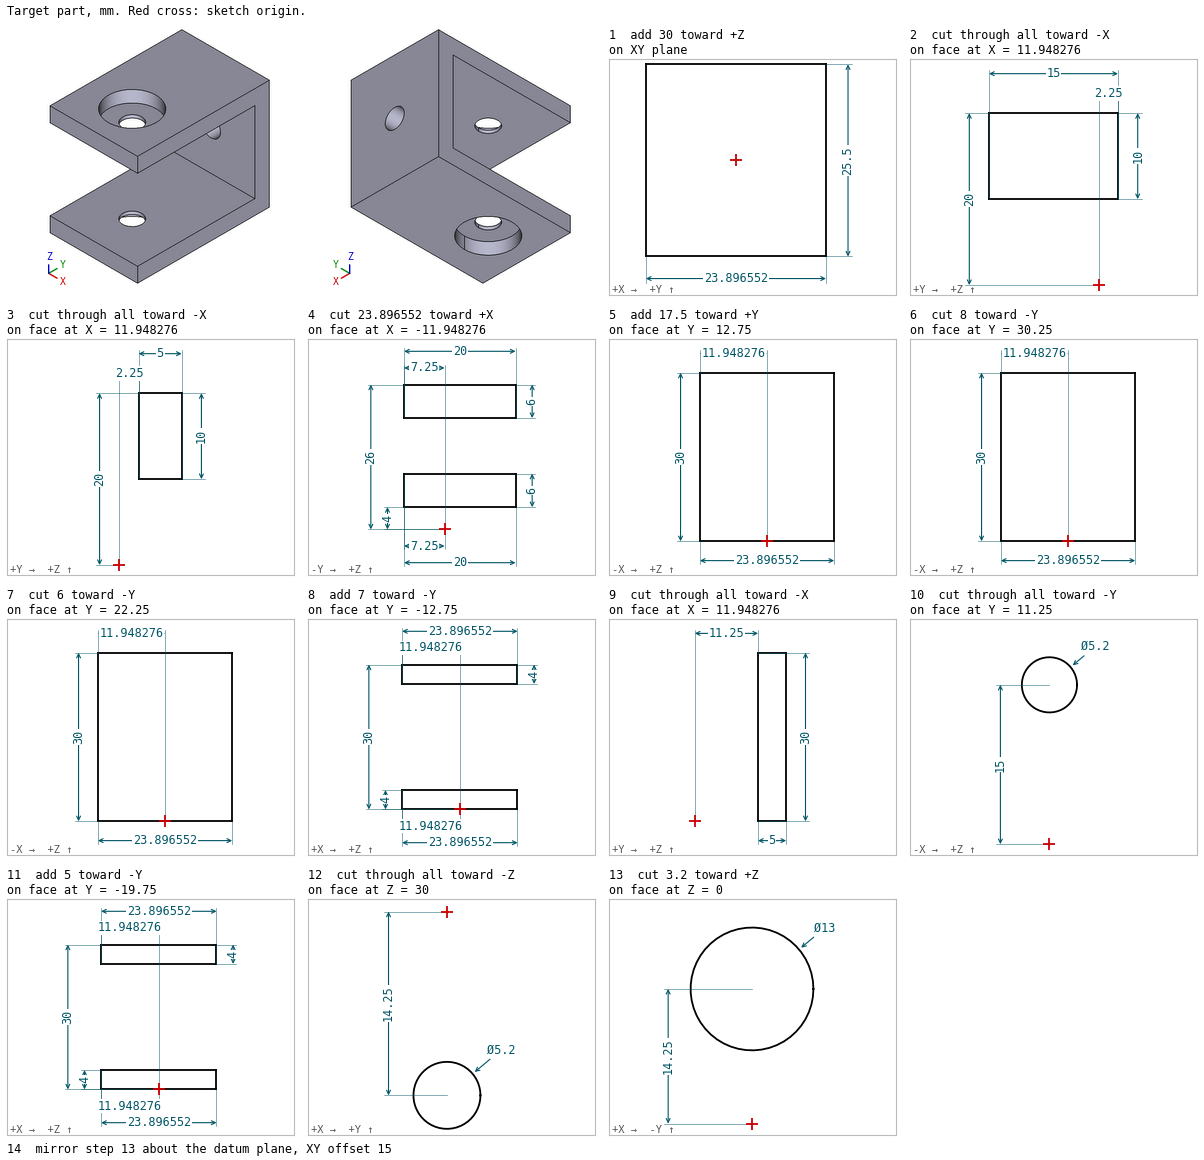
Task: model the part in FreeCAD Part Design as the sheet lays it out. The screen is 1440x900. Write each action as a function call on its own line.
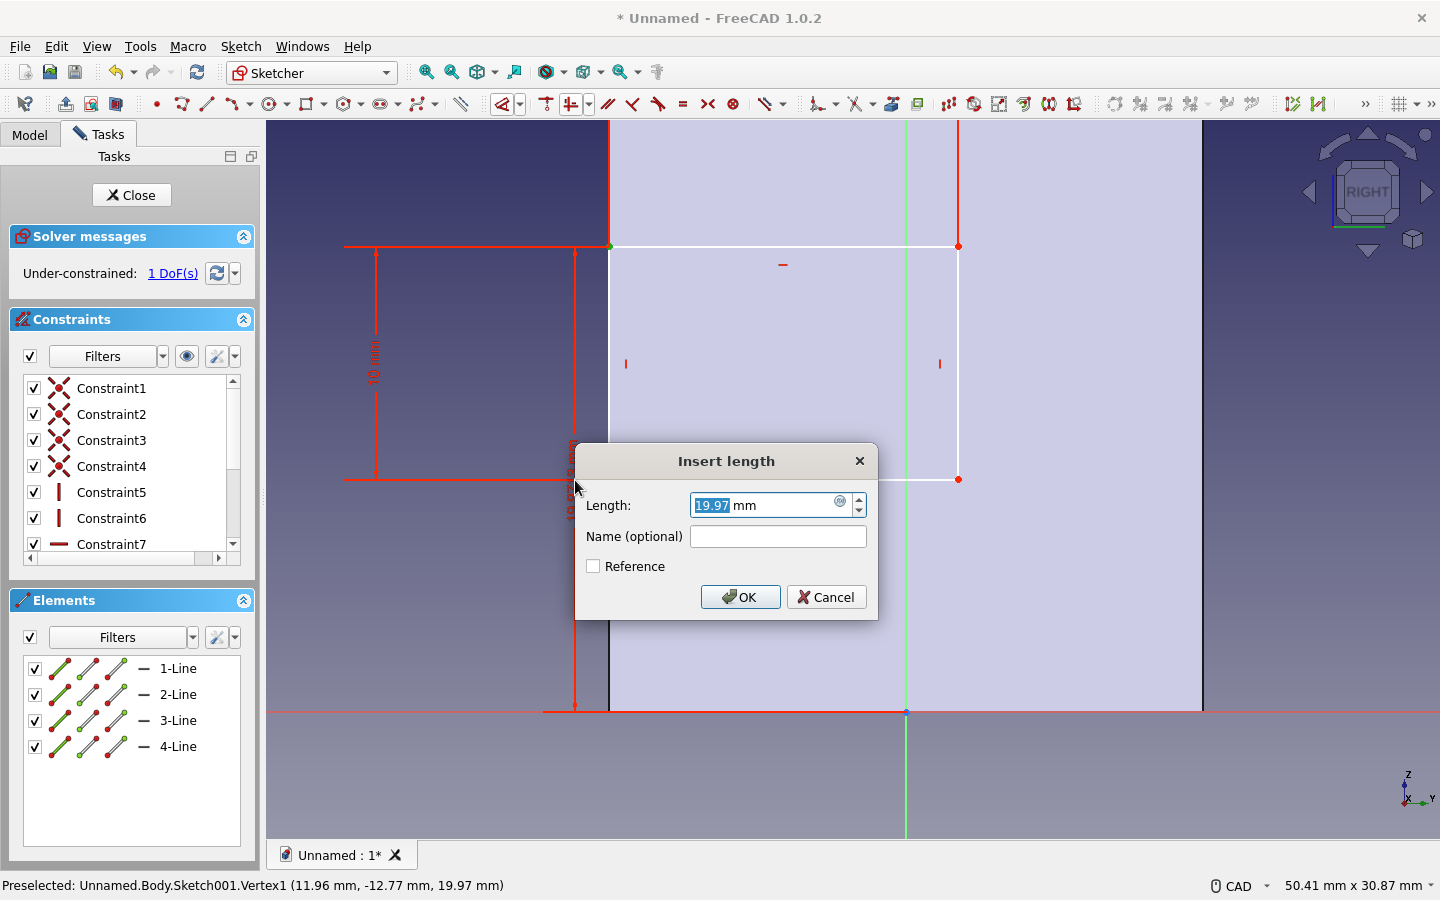
text(20)
key(Return)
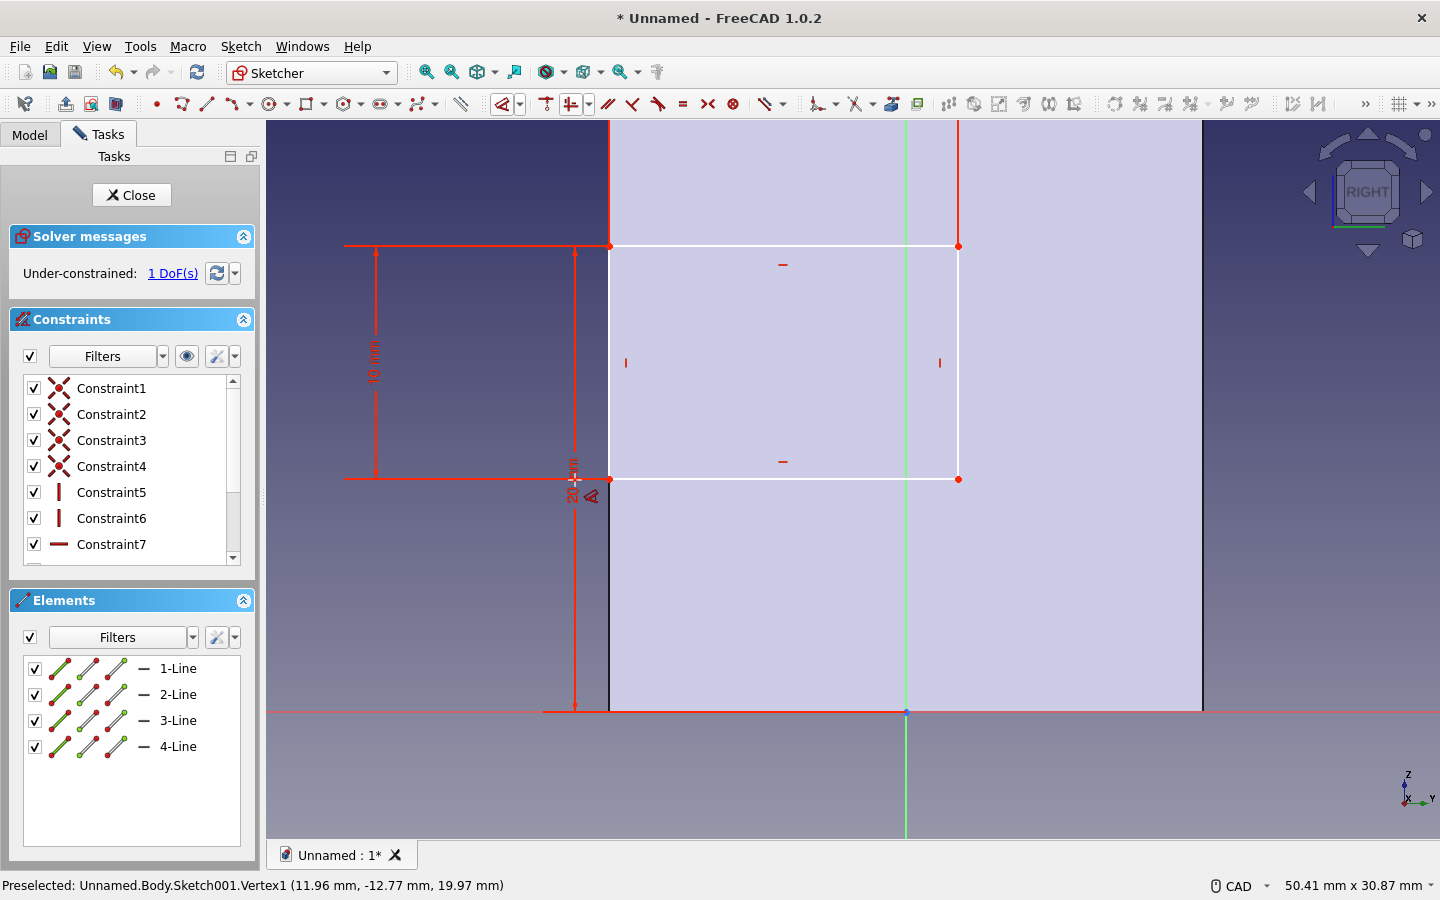
click(958, 479)
click(932, 746)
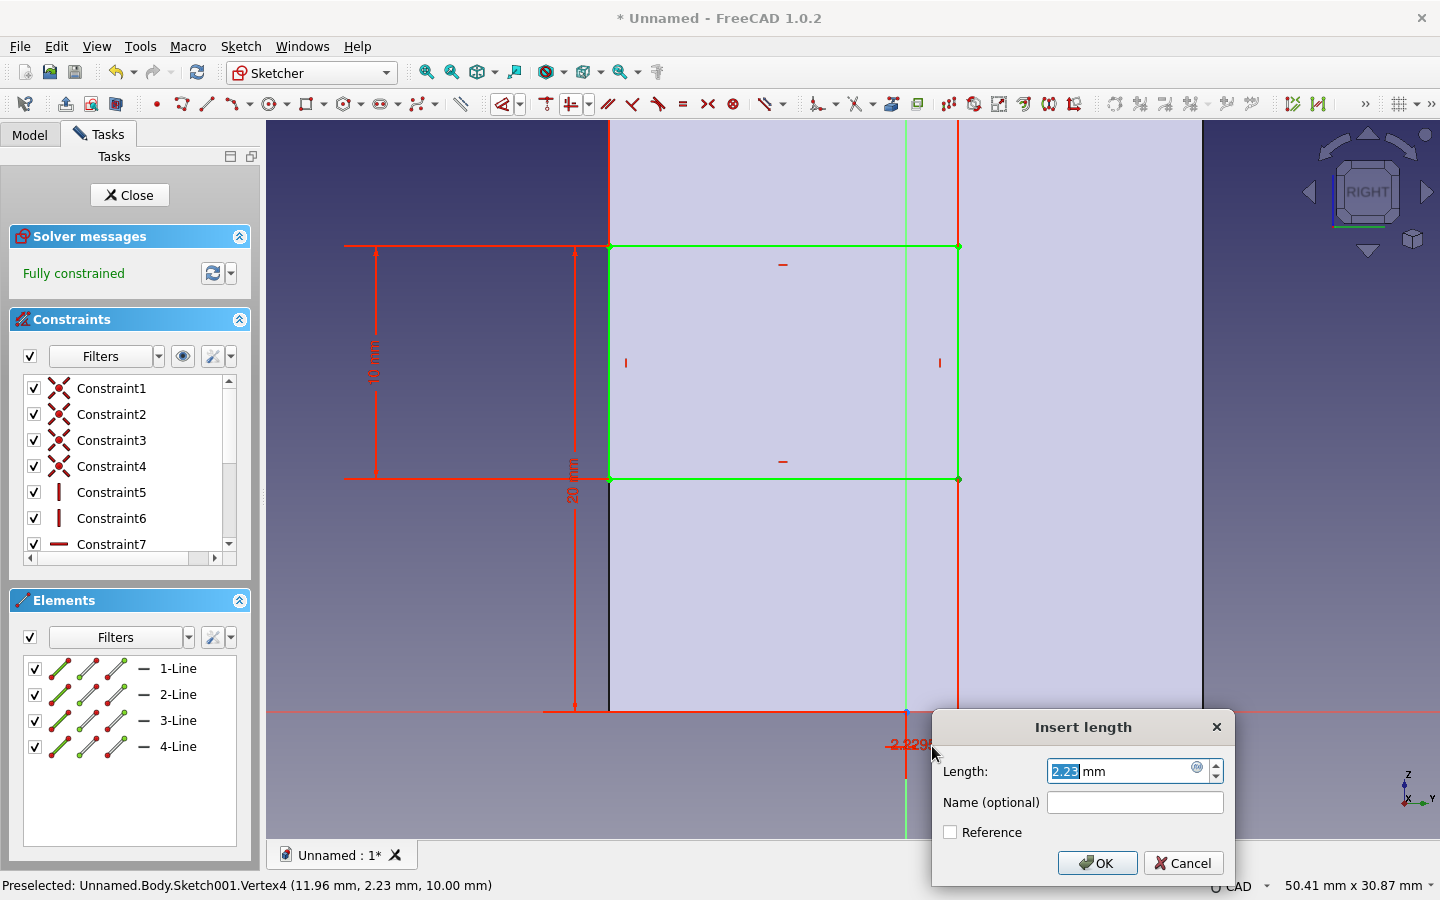
text(2.25)
key(Return)
key(Escape)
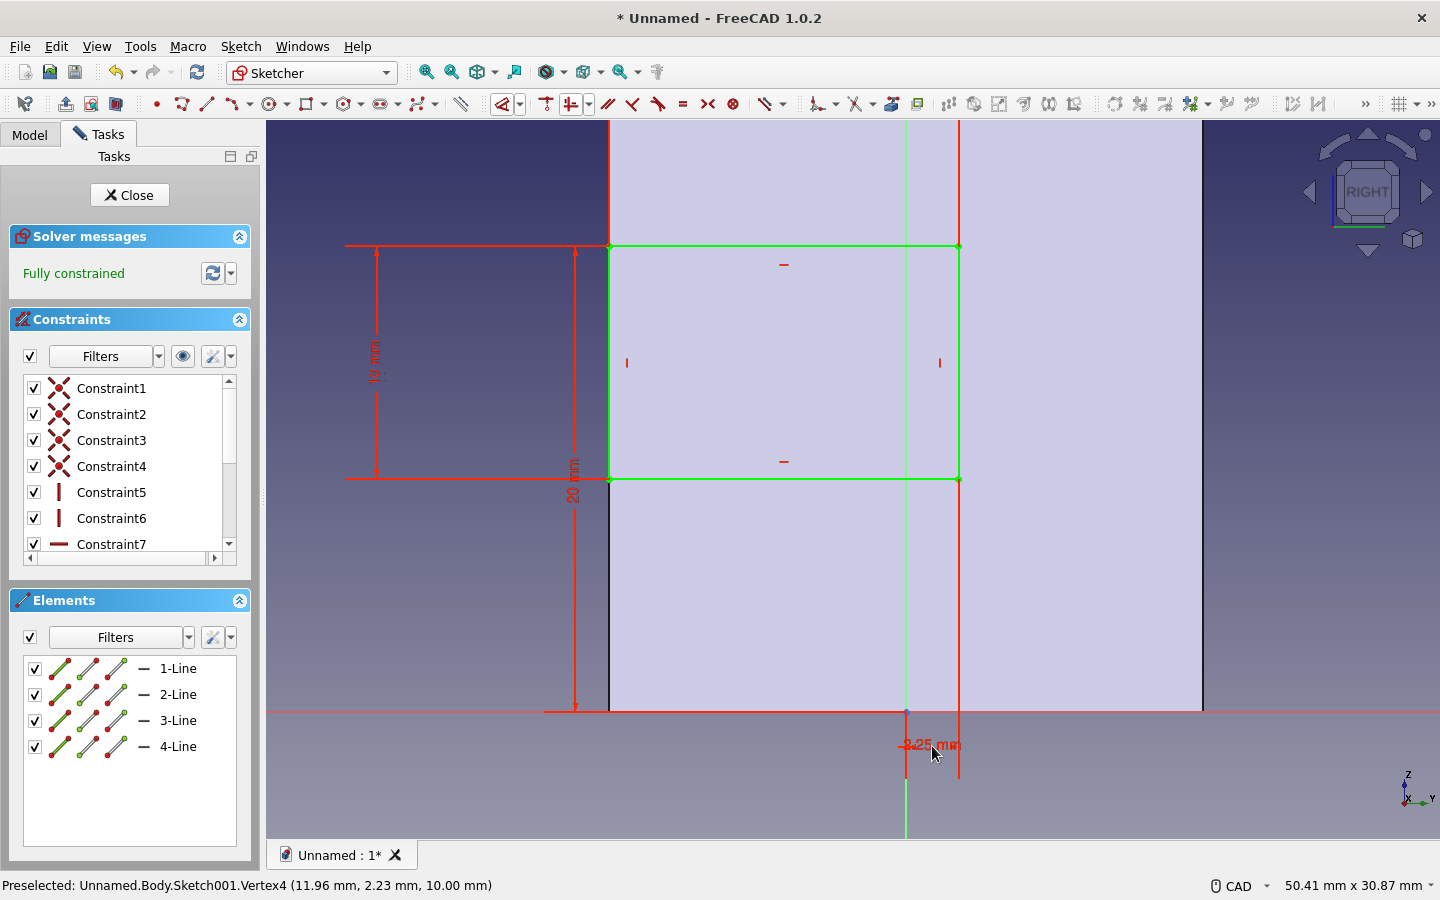
click(130, 195)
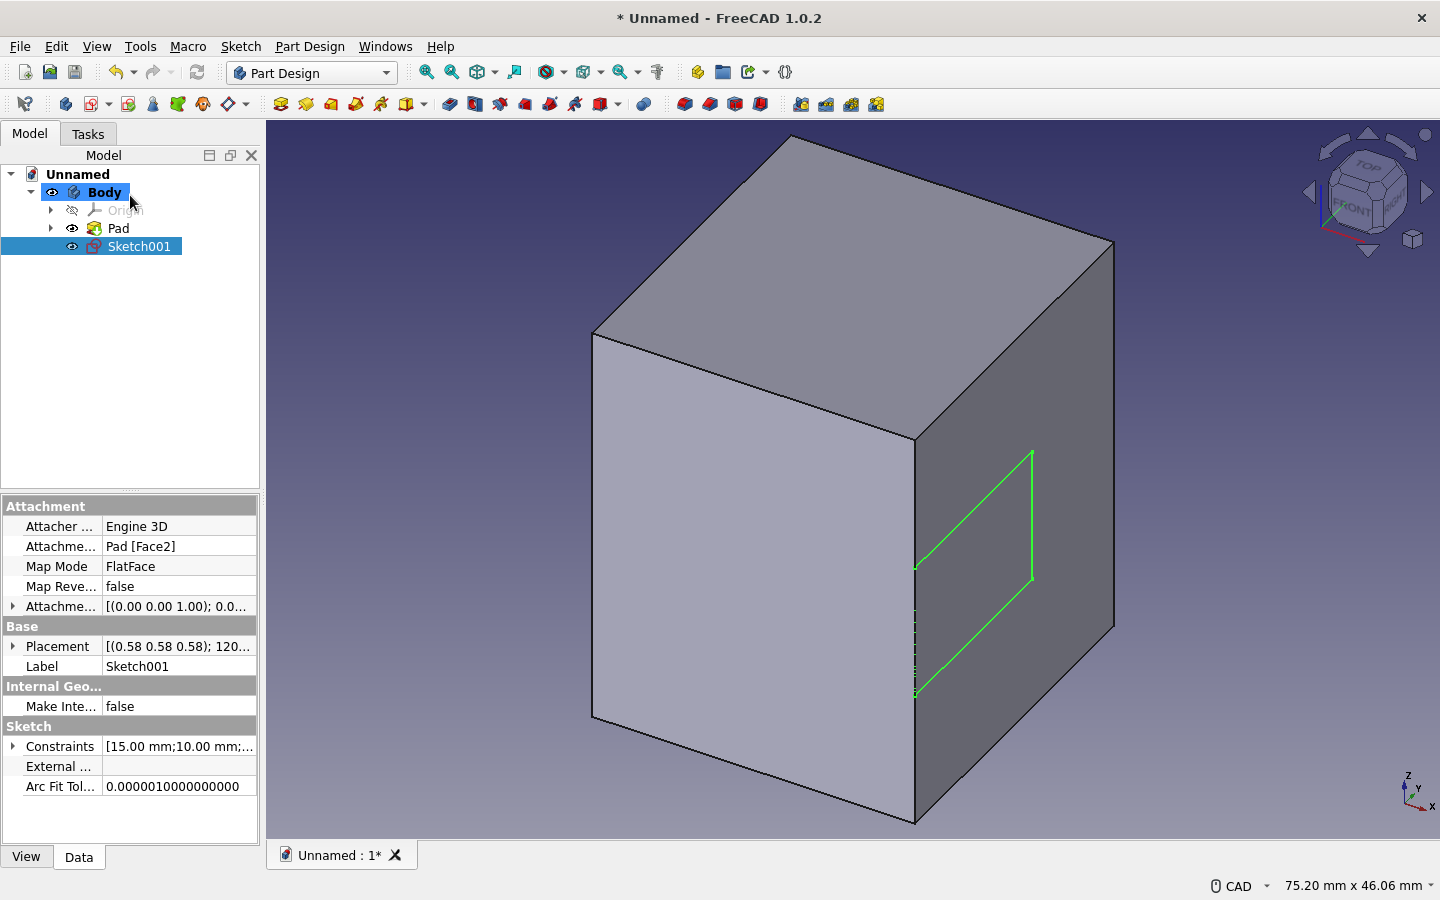
click(450, 104)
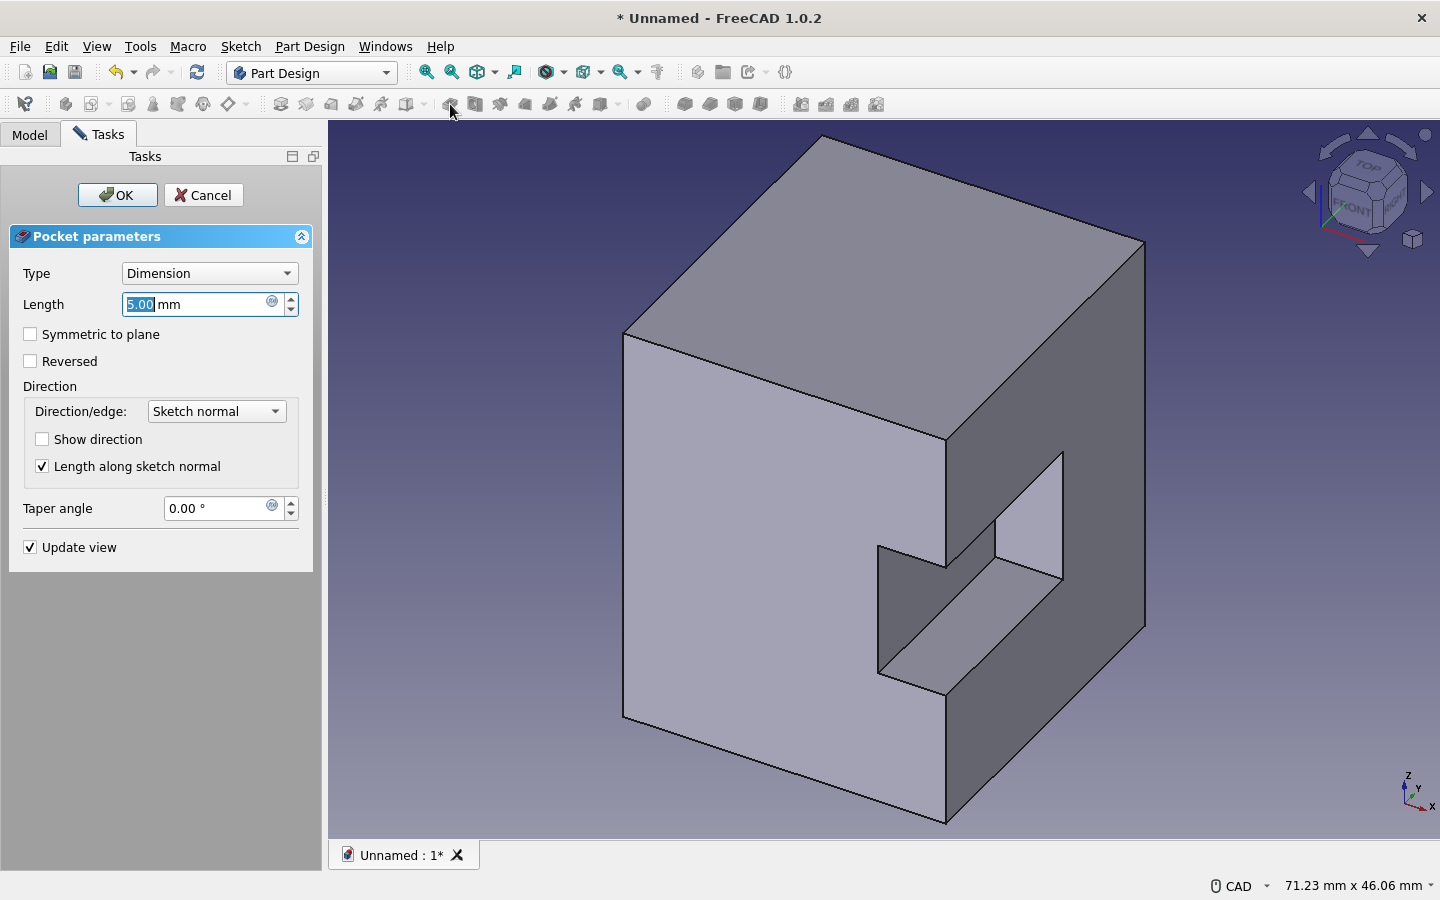
click(210, 274)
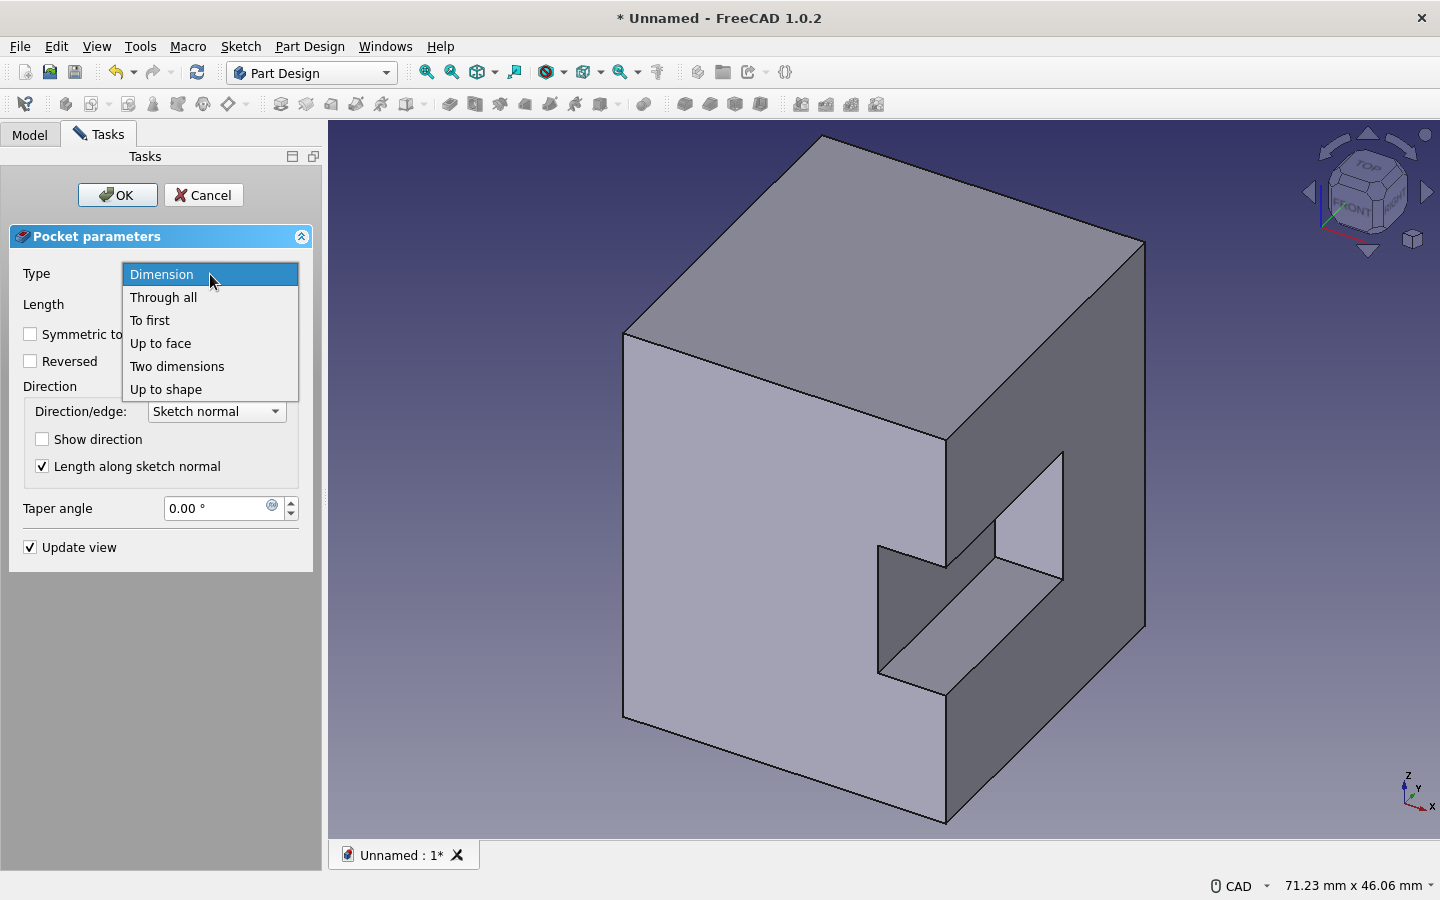
click(208, 298)